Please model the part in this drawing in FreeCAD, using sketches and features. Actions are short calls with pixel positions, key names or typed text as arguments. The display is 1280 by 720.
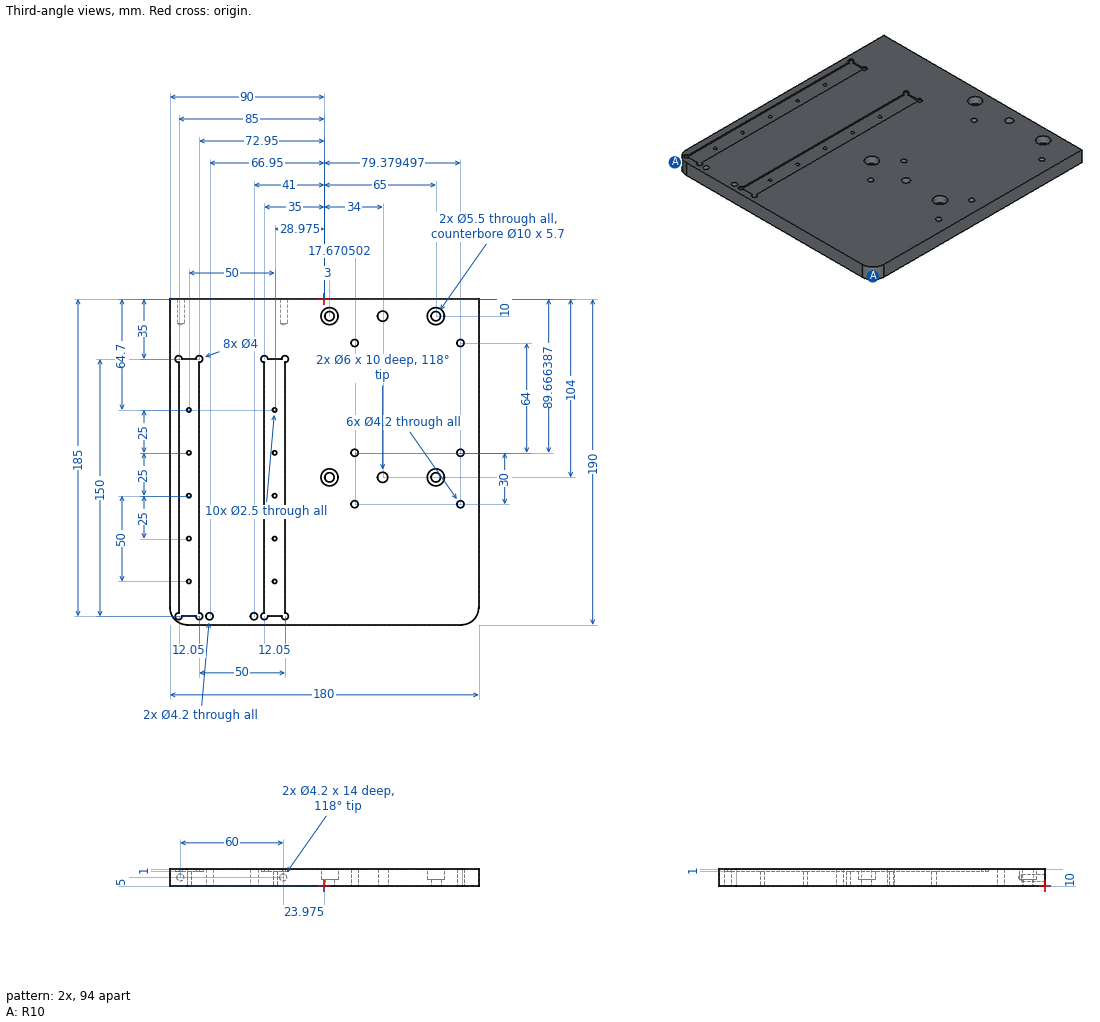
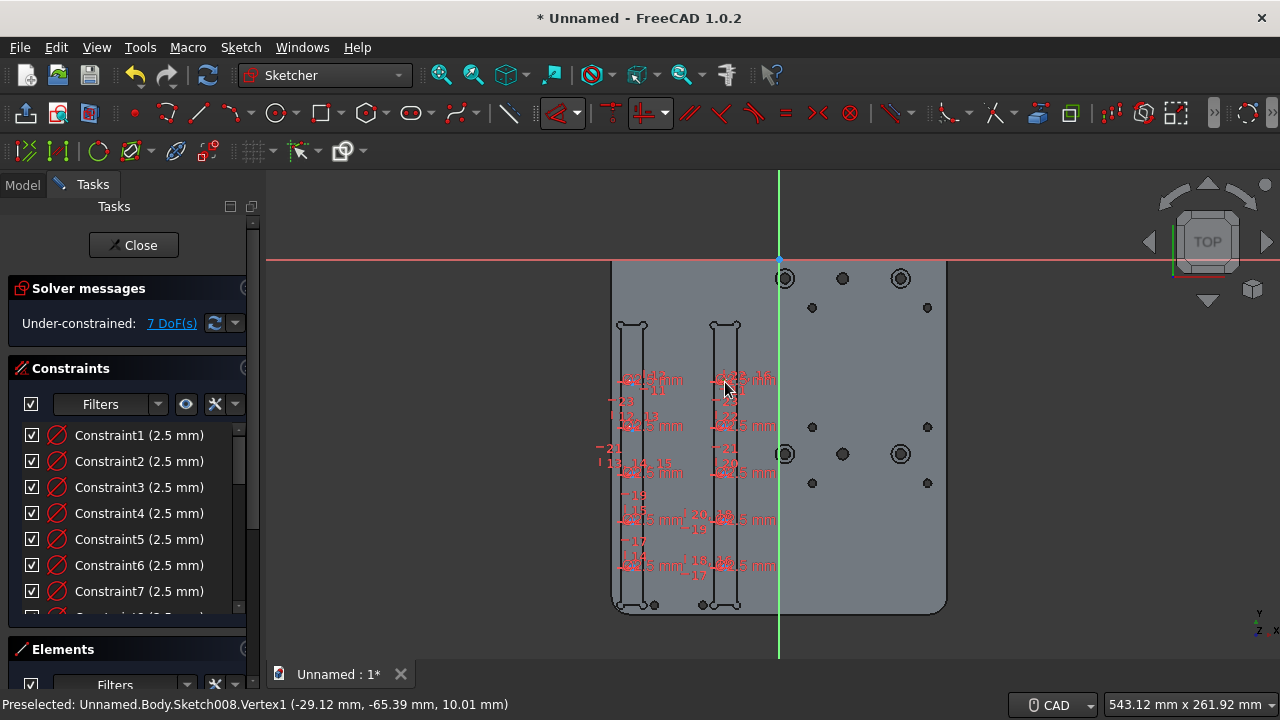
click(632, 382)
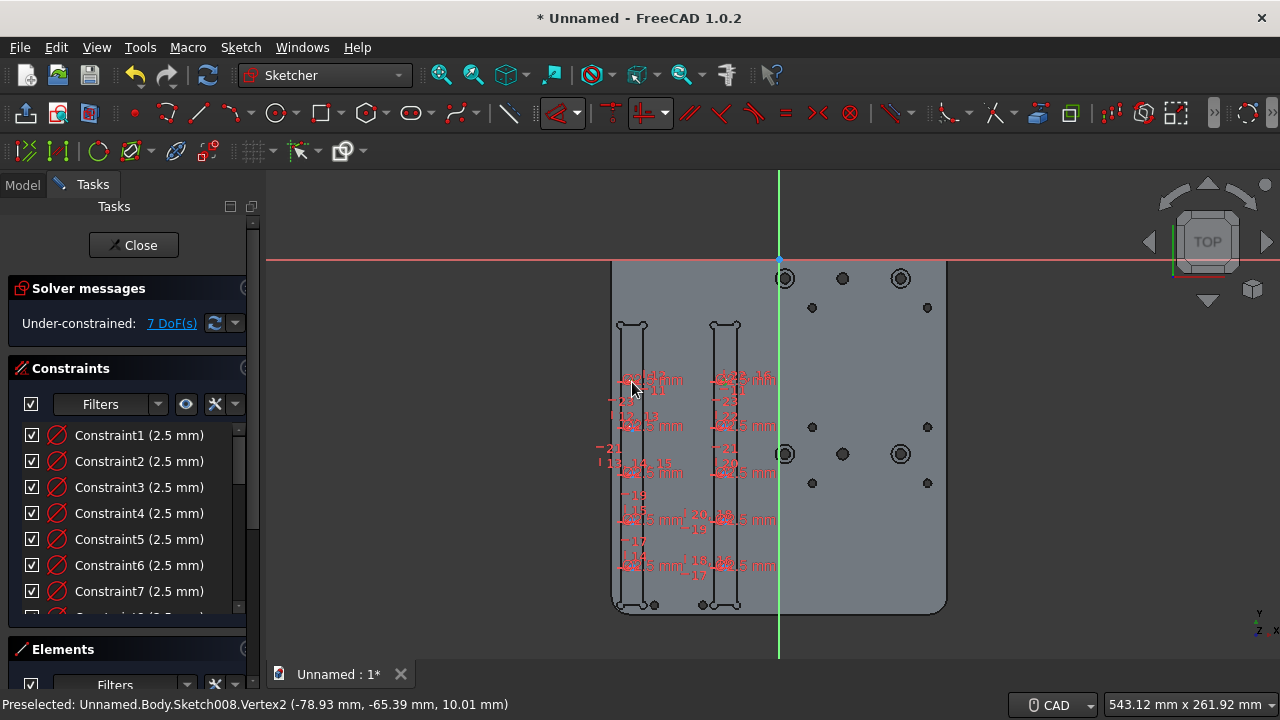
key(l)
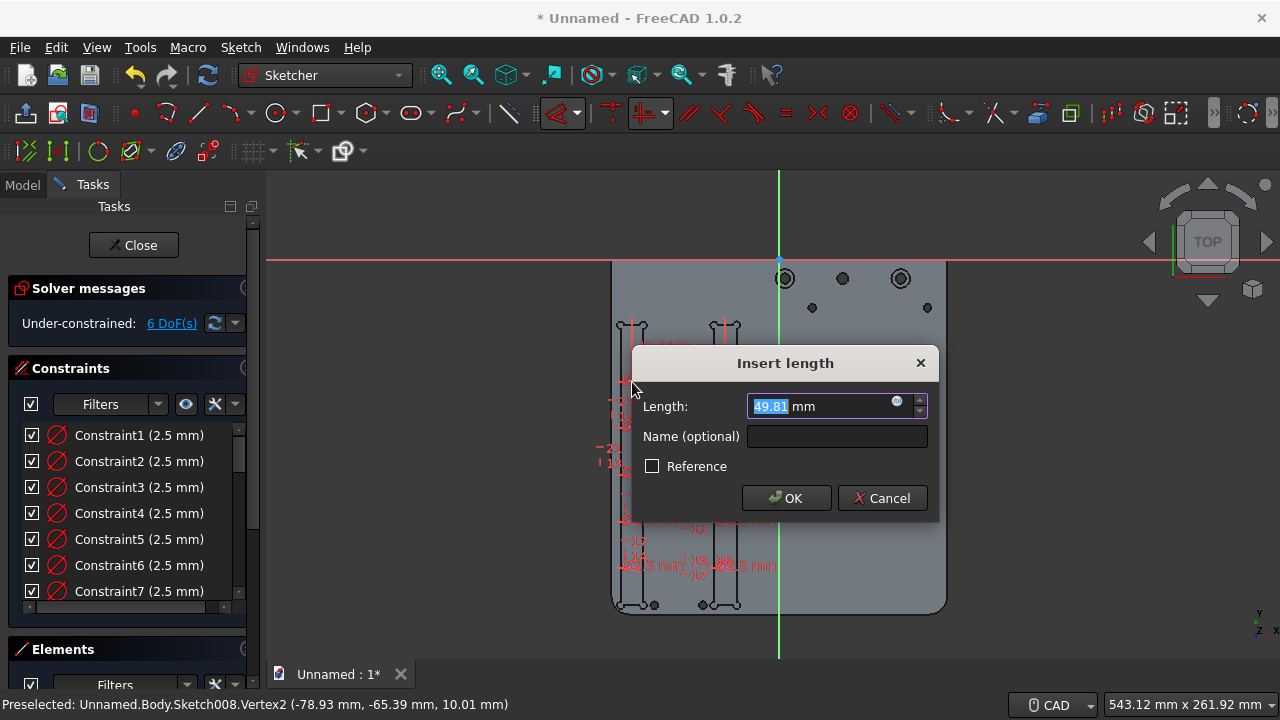
text(50)
key(Return)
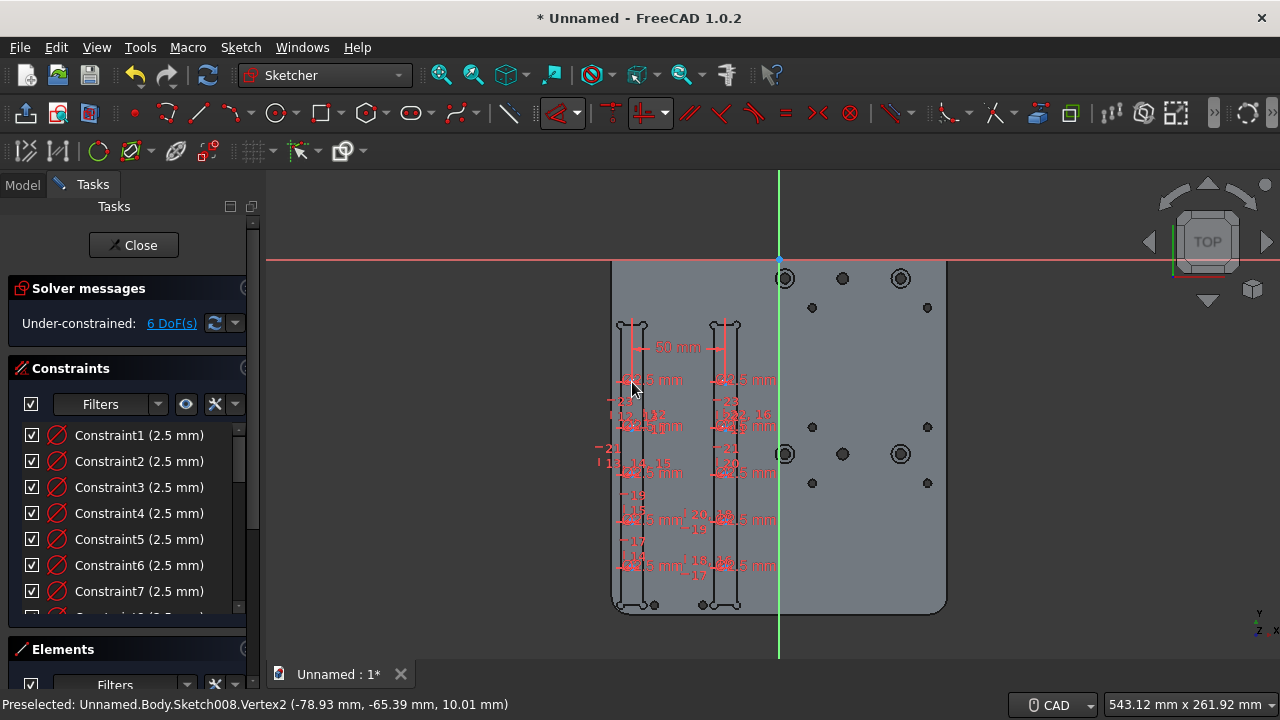
click(632, 382)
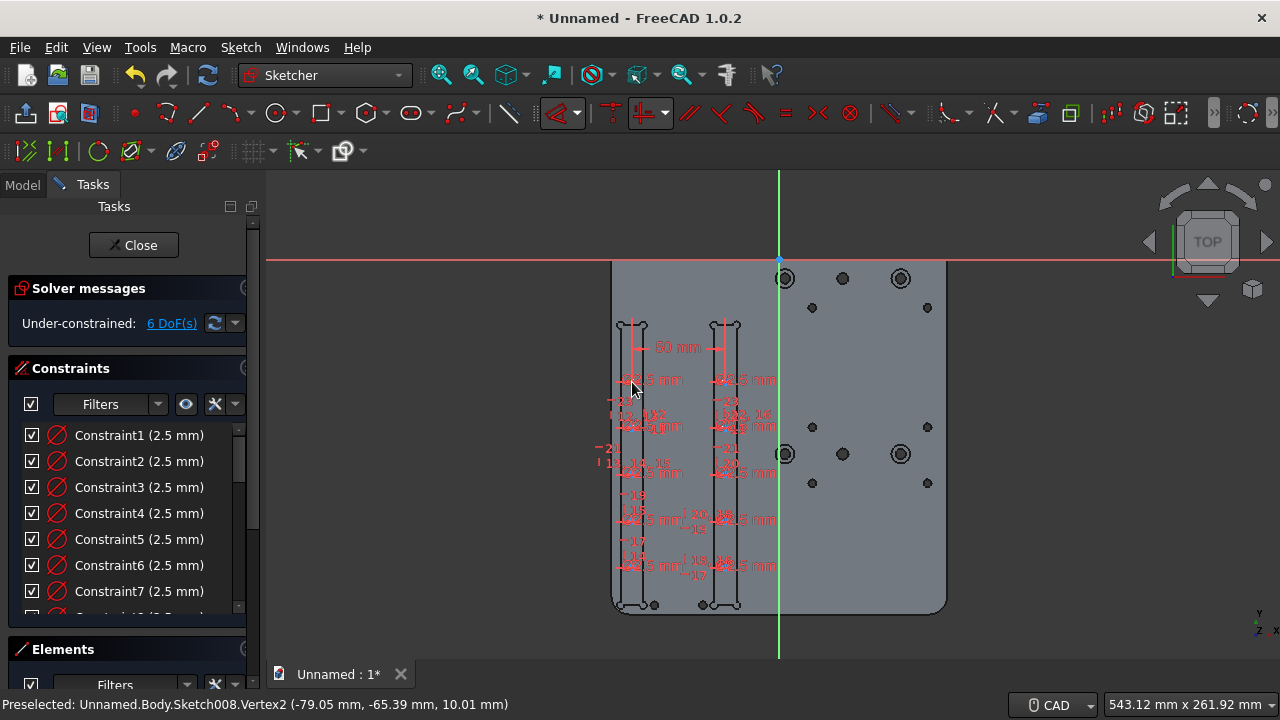
click(632, 428)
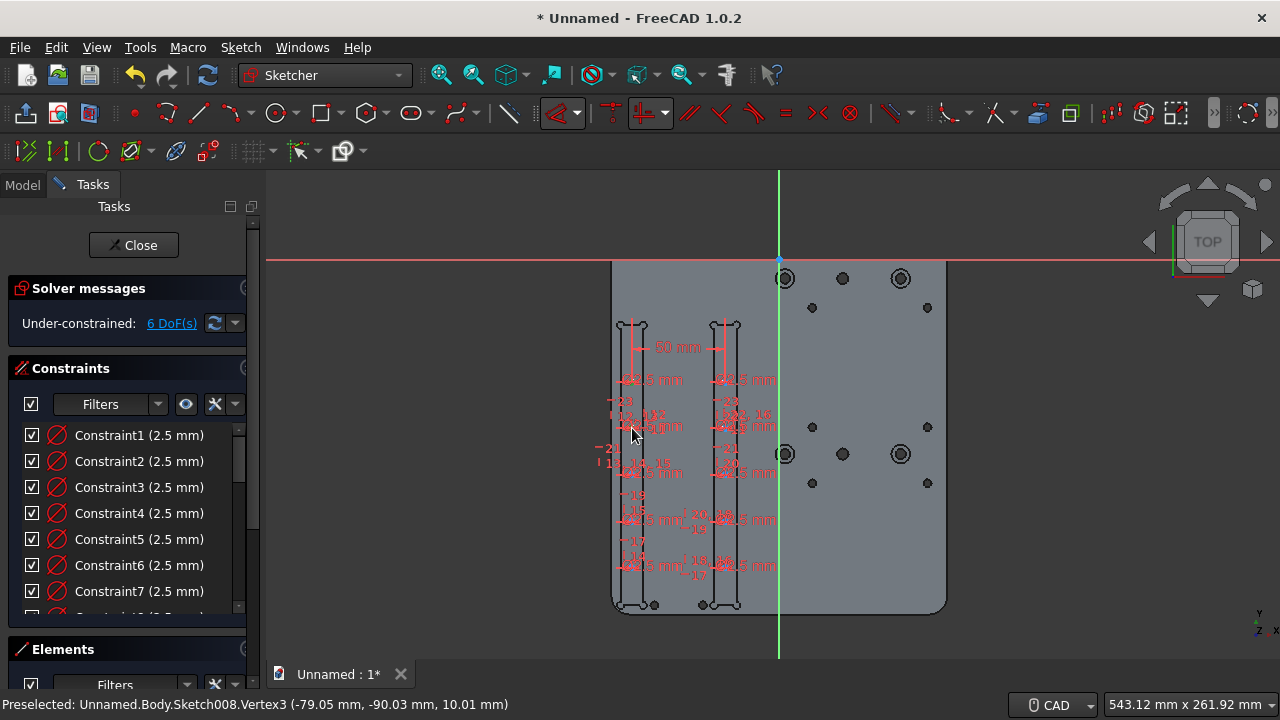
click(580, 114)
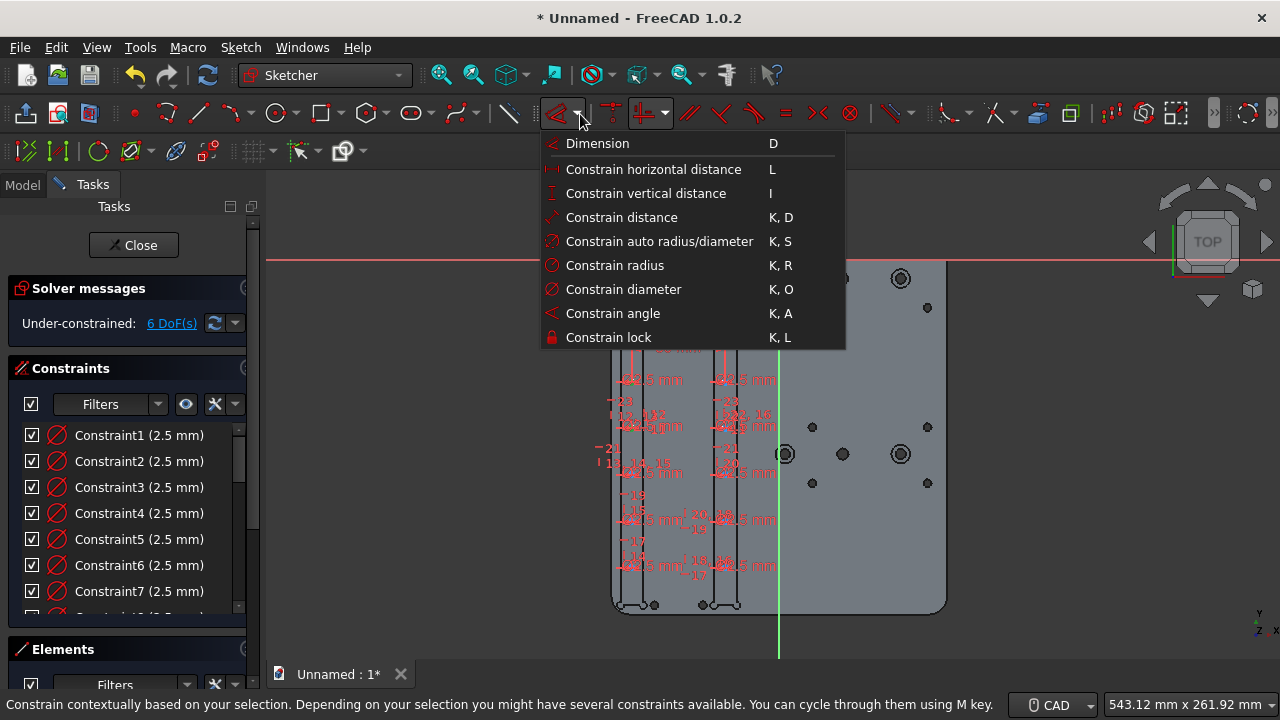
click(693, 193)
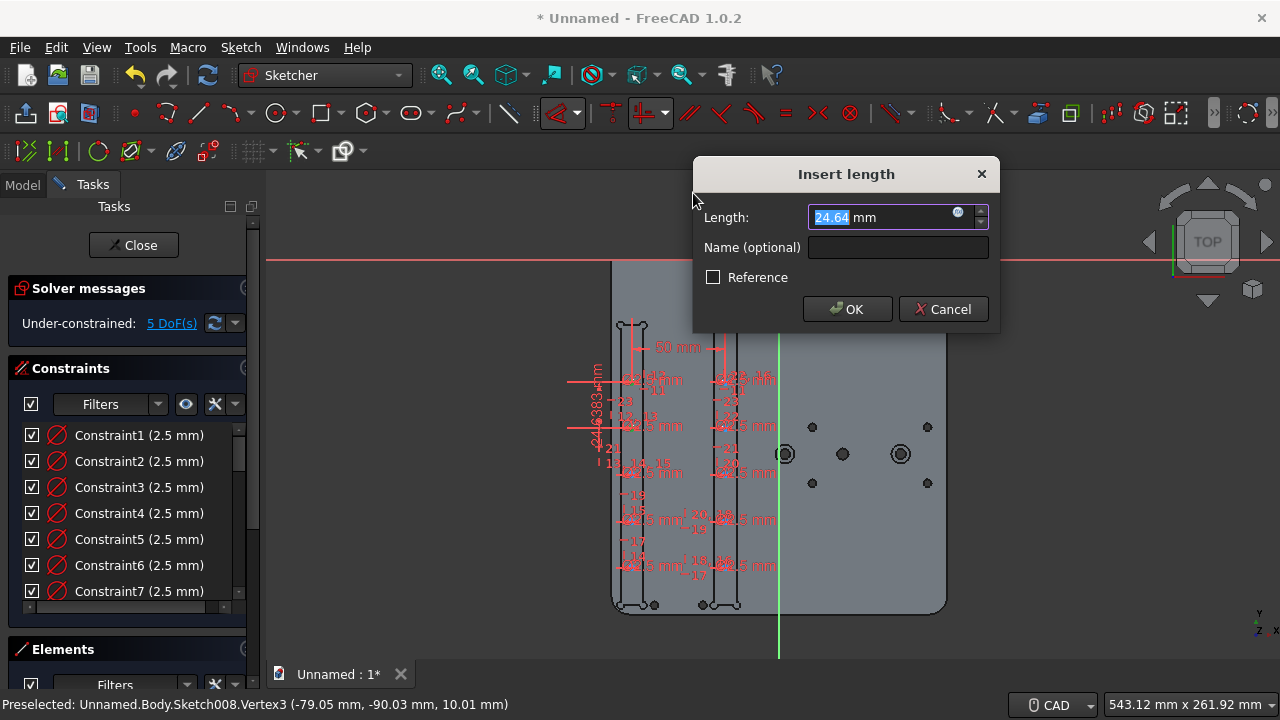
text(25)
key(Return)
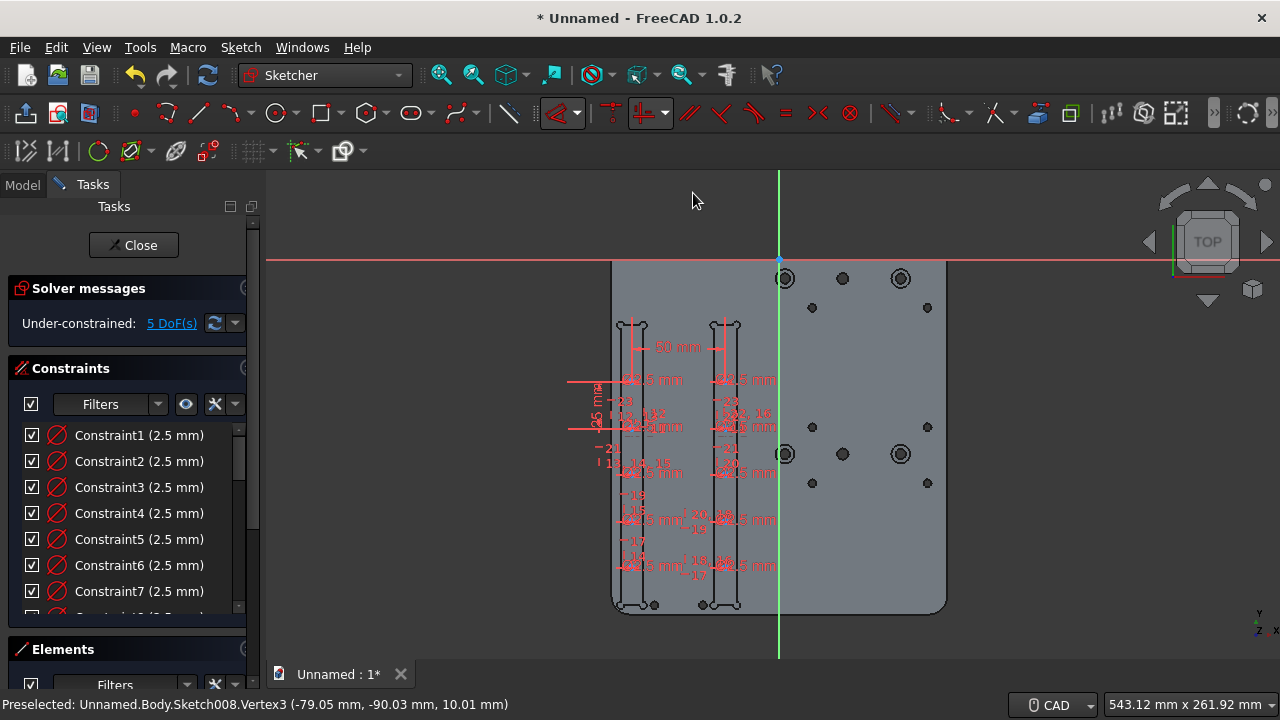
click(632, 429)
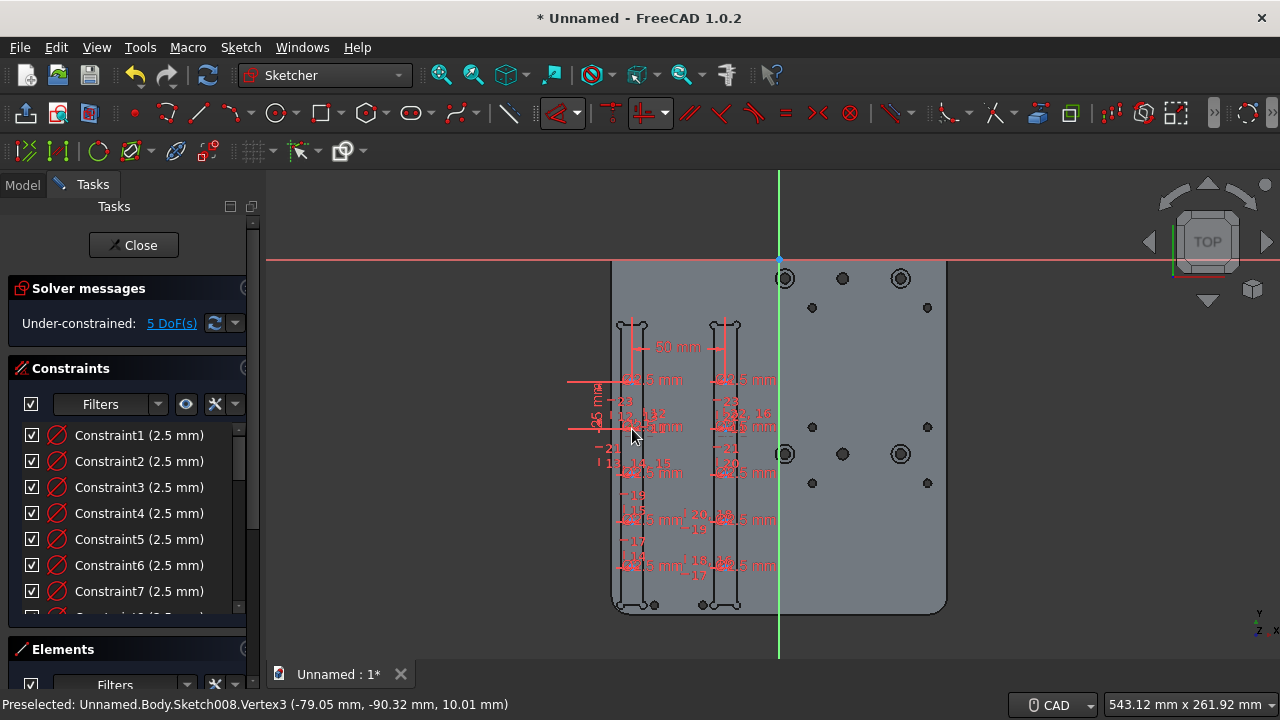
click(632, 475)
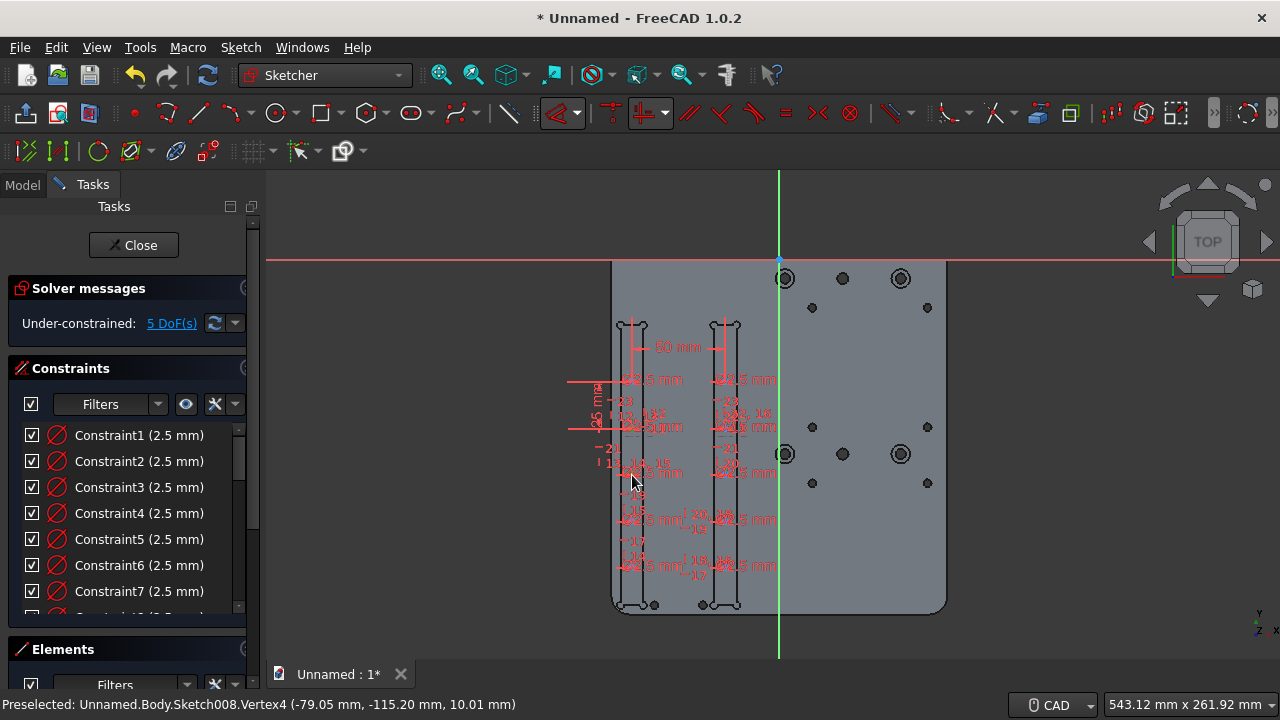
key(i)